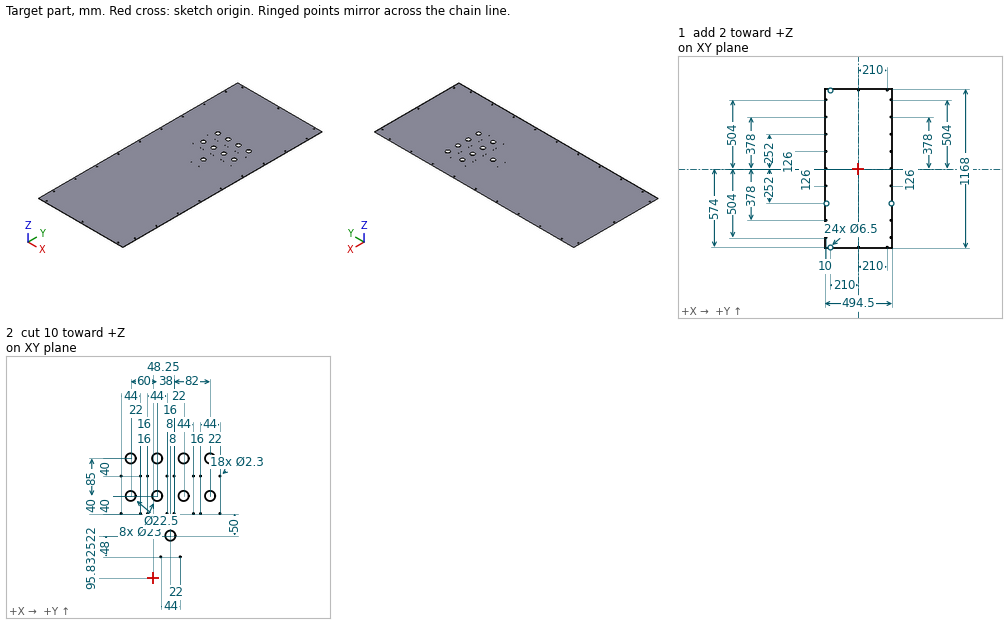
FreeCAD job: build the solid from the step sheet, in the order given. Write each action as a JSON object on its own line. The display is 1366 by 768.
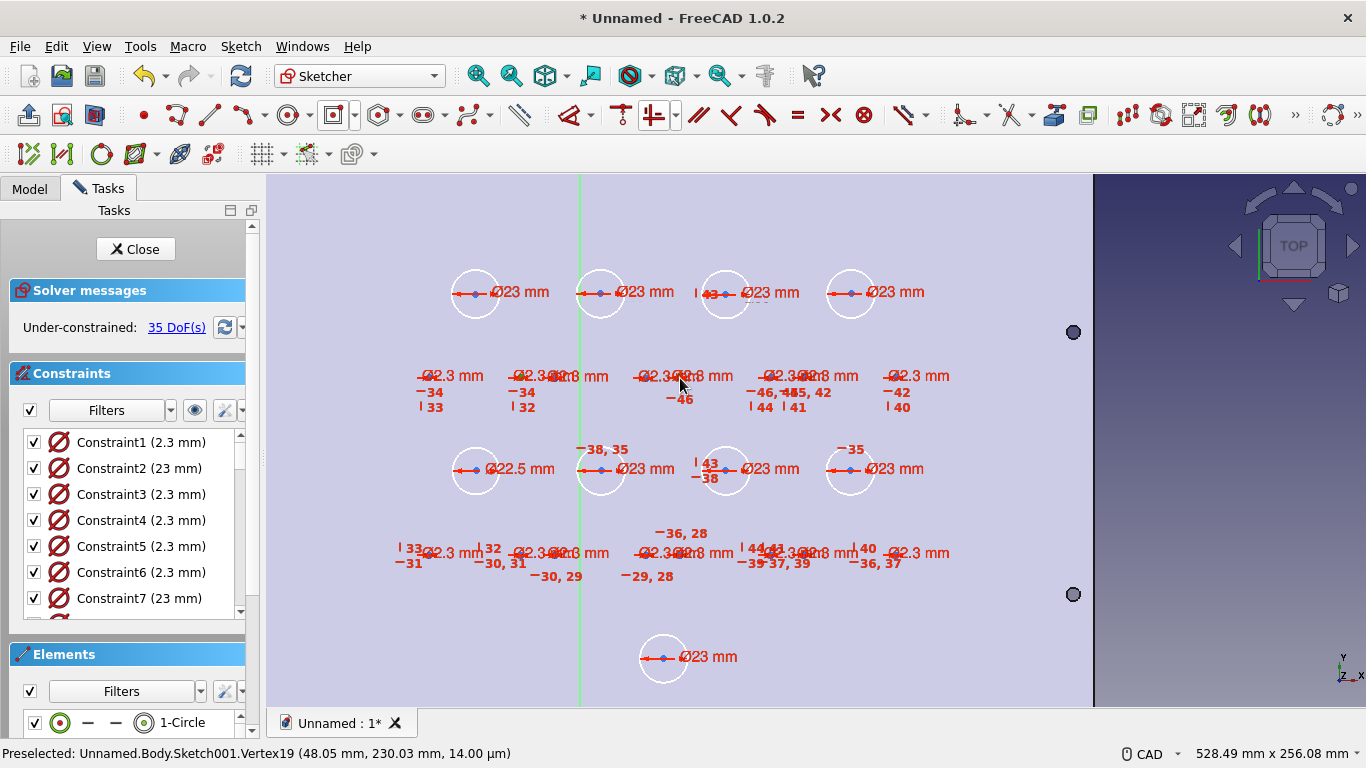
{"action": "left_click", "coordinate": [676, 116]}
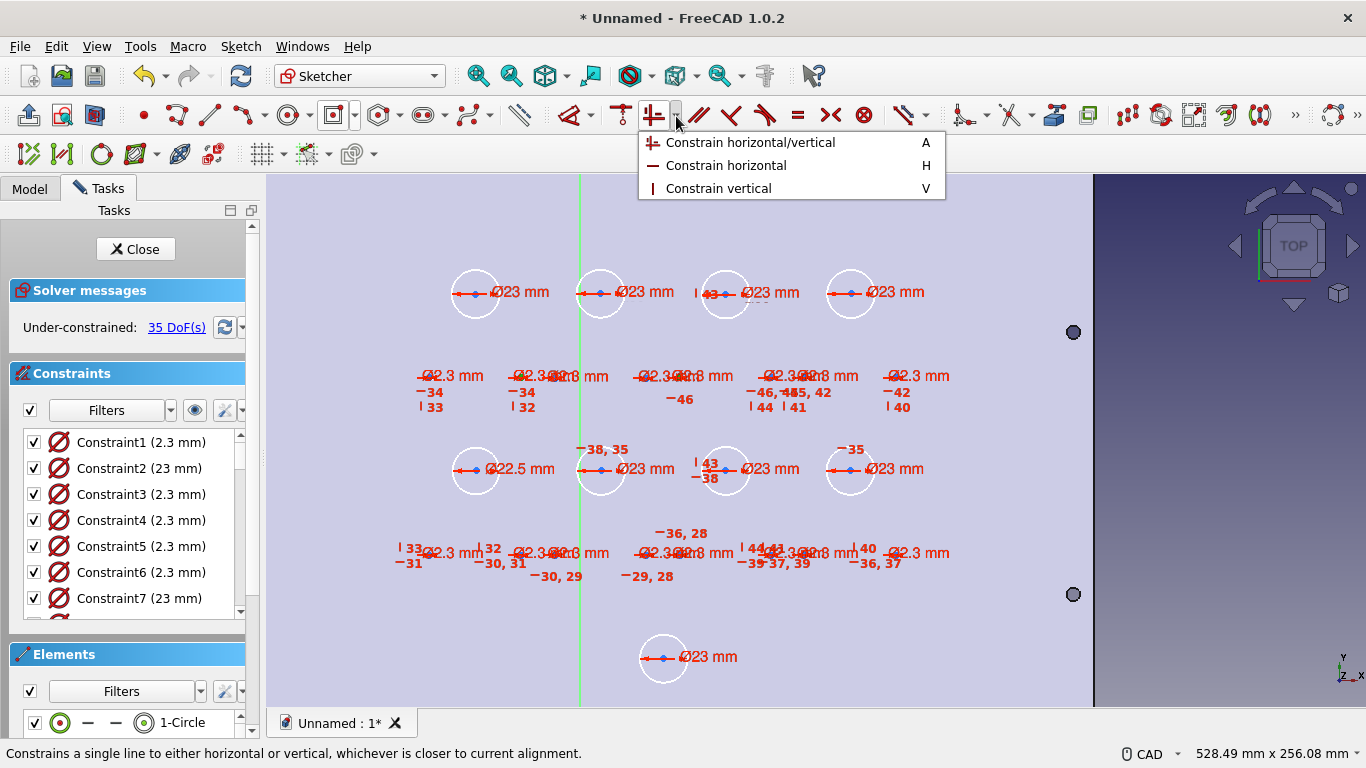
{"action": "left_click", "coordinate": [792, 166]}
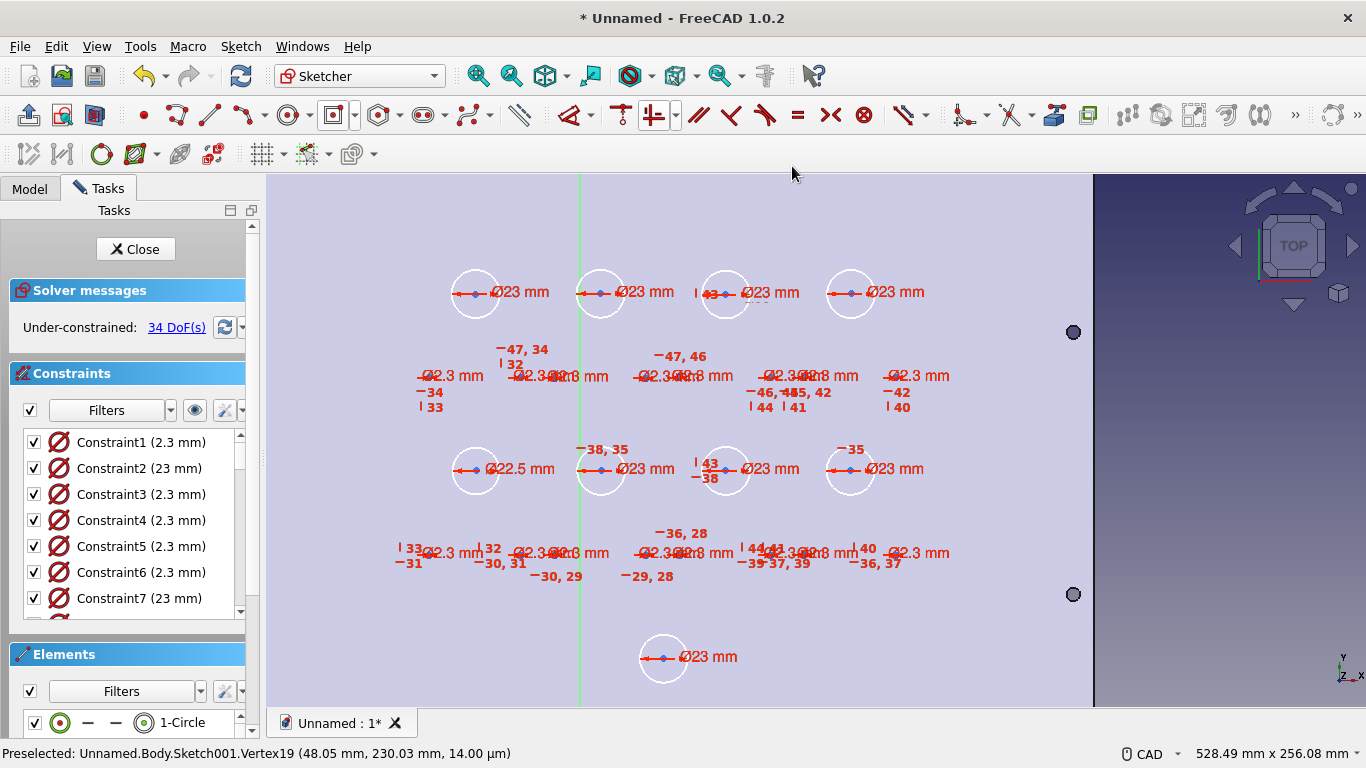
{"action": "left_click", "coordinate": [601, 471]}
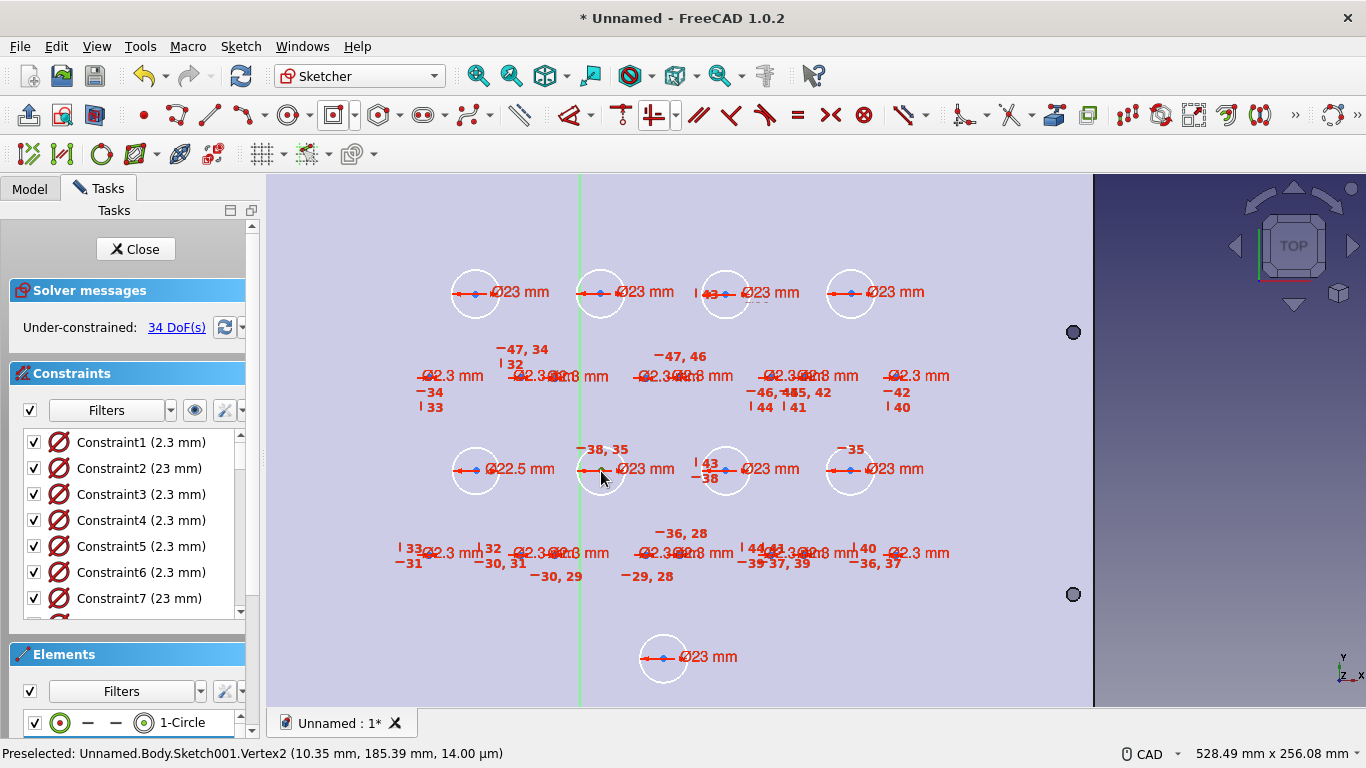
{"action": "left_click", "coordinate": [601, 294]}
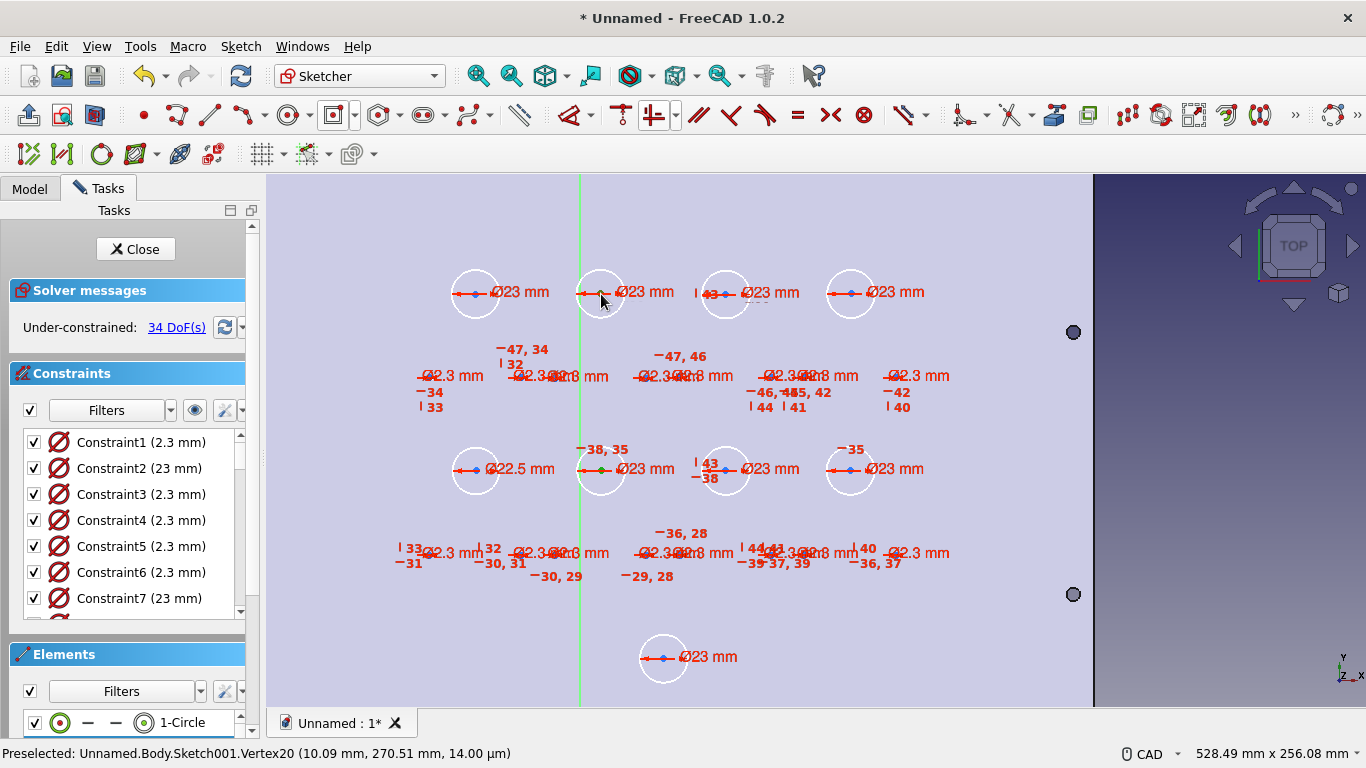
{"action": "key", "text": "v"}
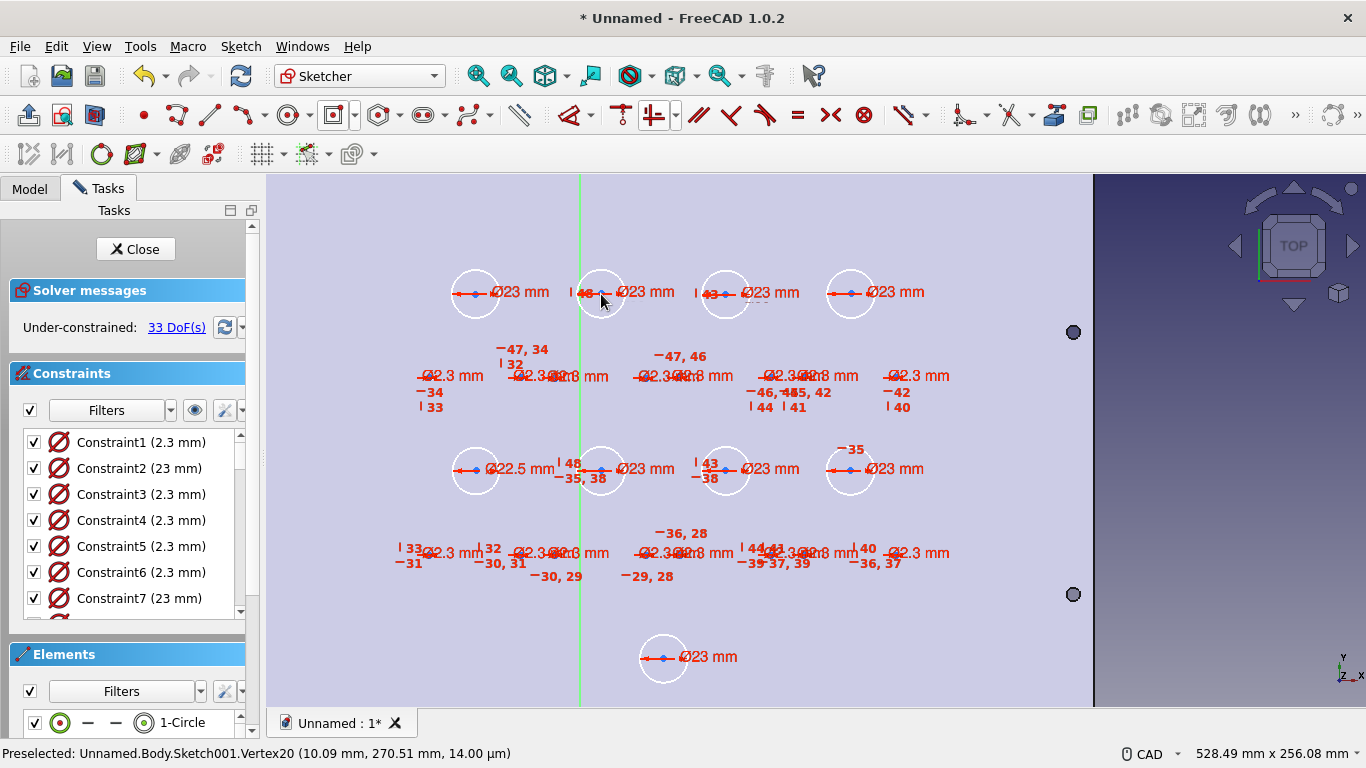
{"action": "left_click", "coordinate": [476, 294]}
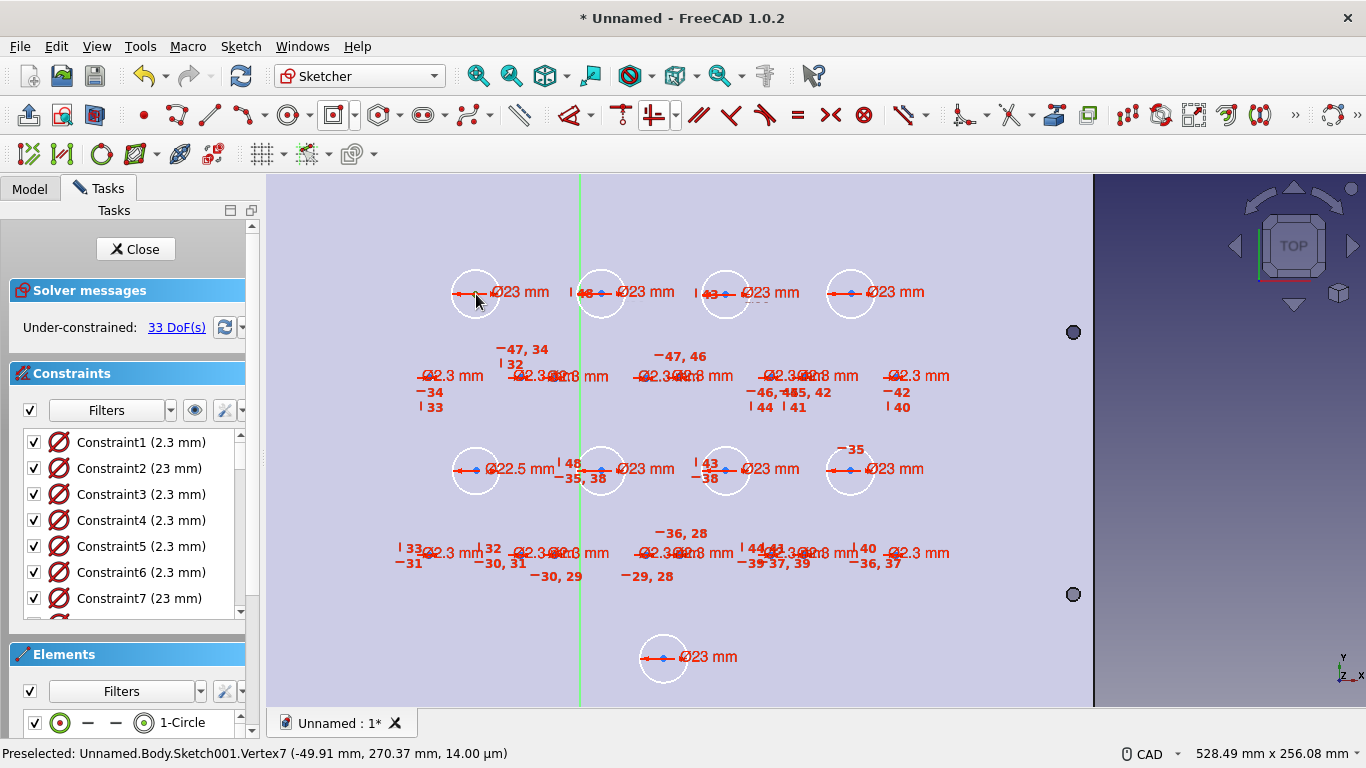
{"action": "left_click", "coordinate": [601, 294]}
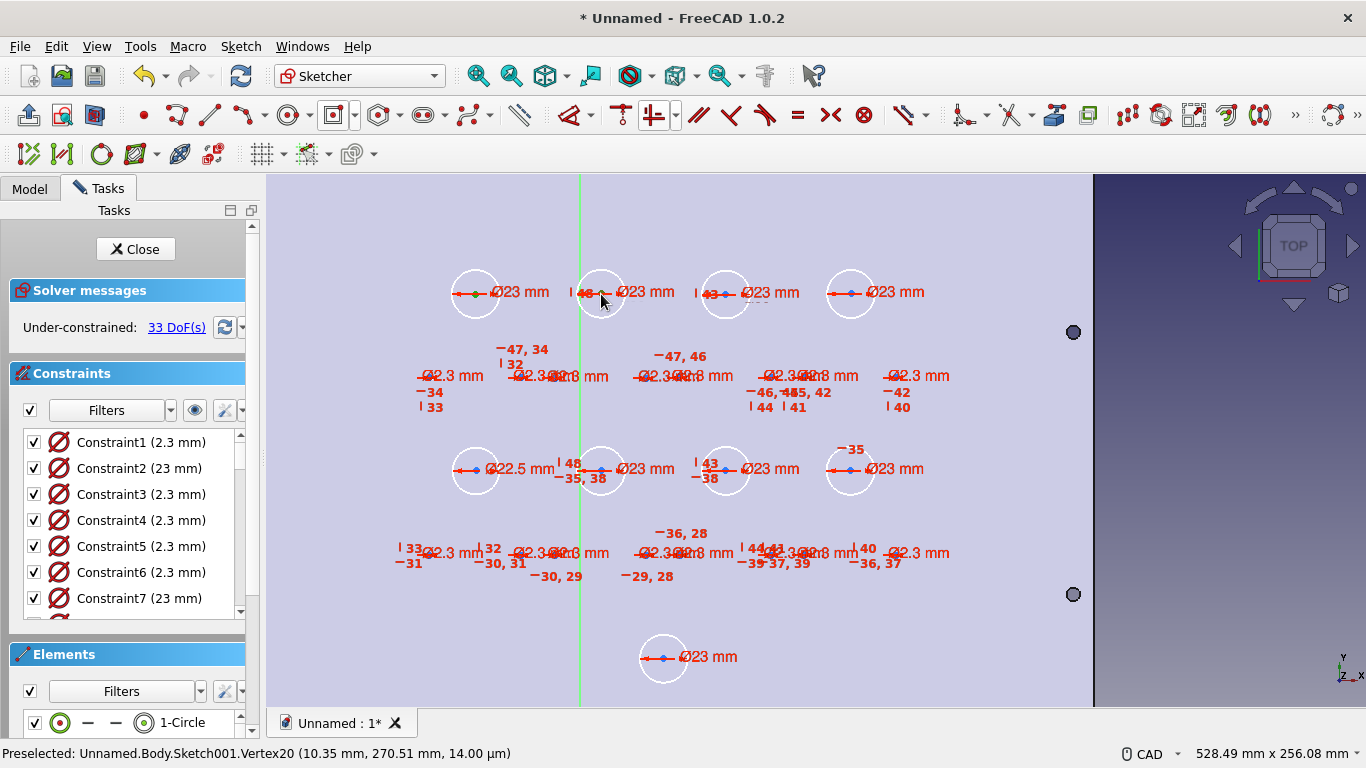
{"action": "key", "text": "h"}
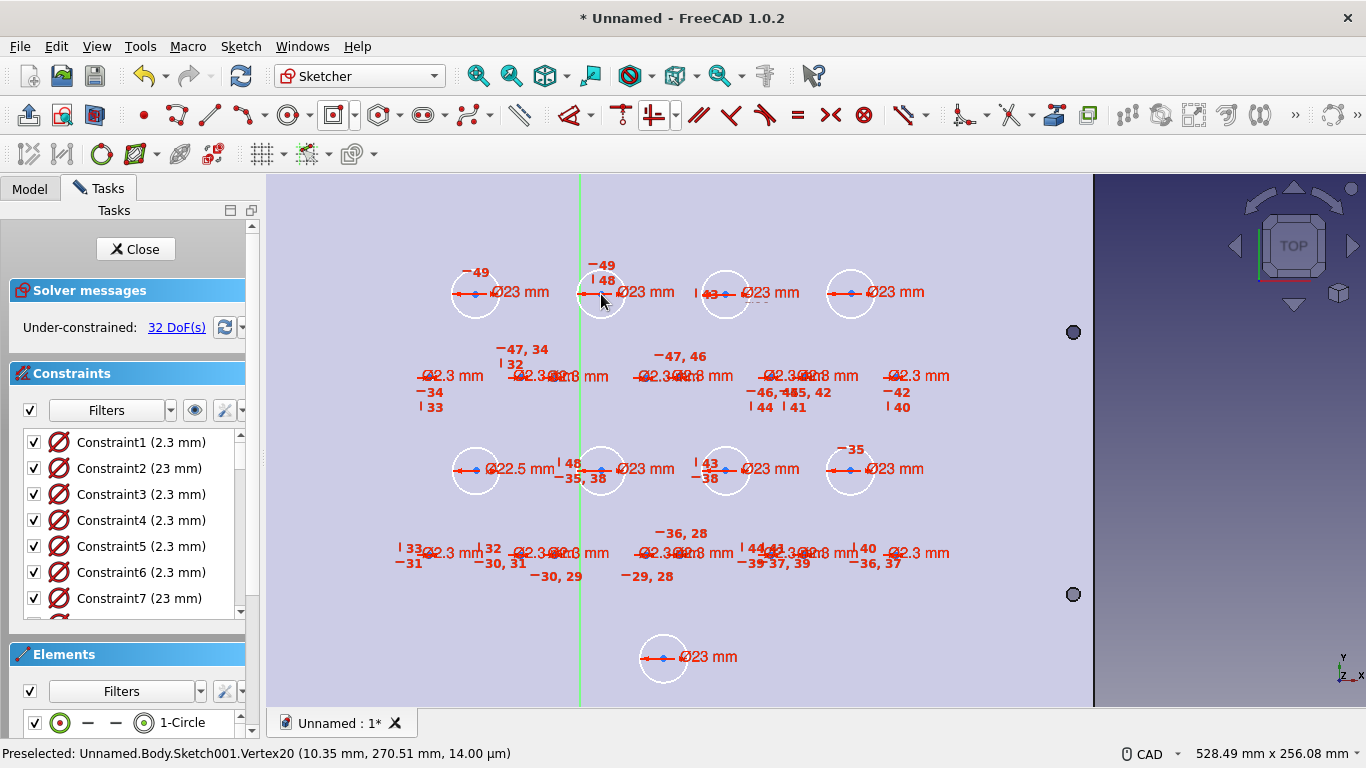
{"action": "left_click", "coordinate": [726, 295]}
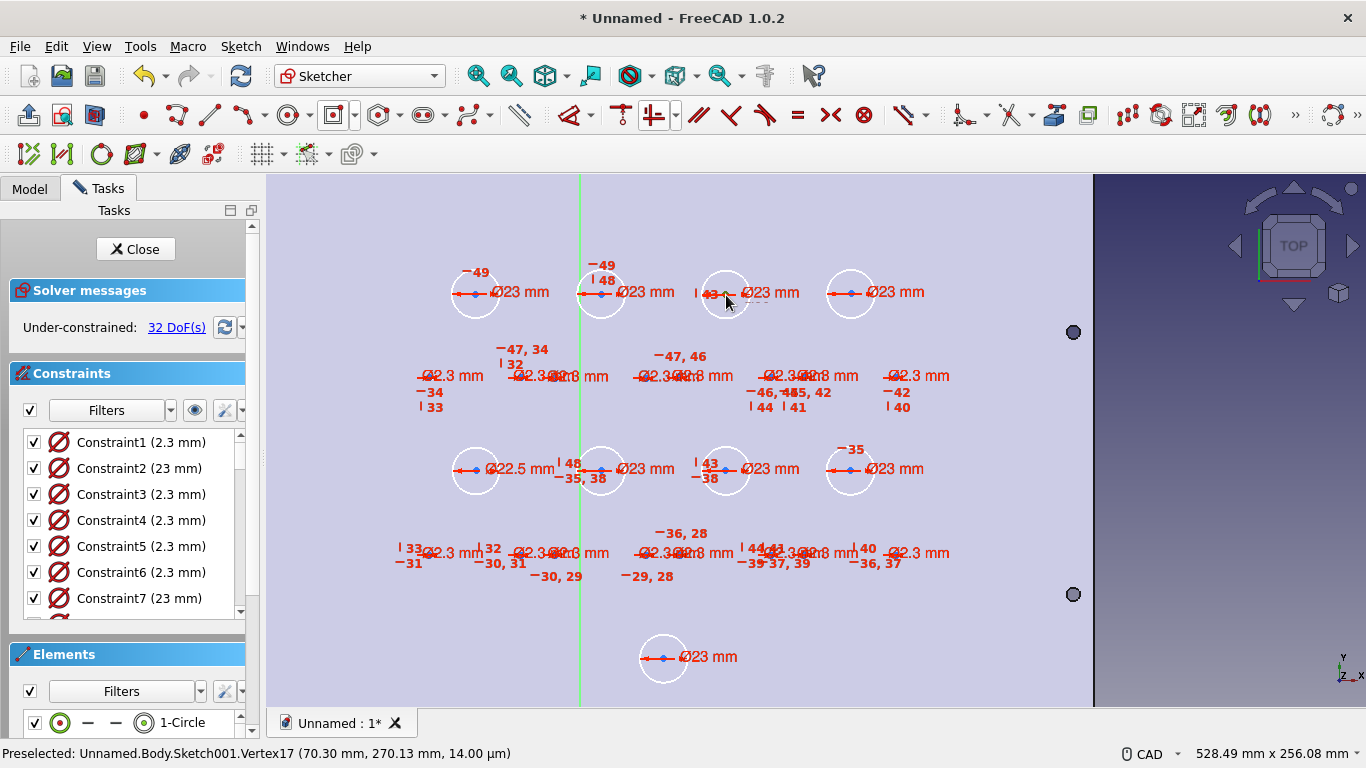
{"action": "left_click", "coordinate": [601, 294]}